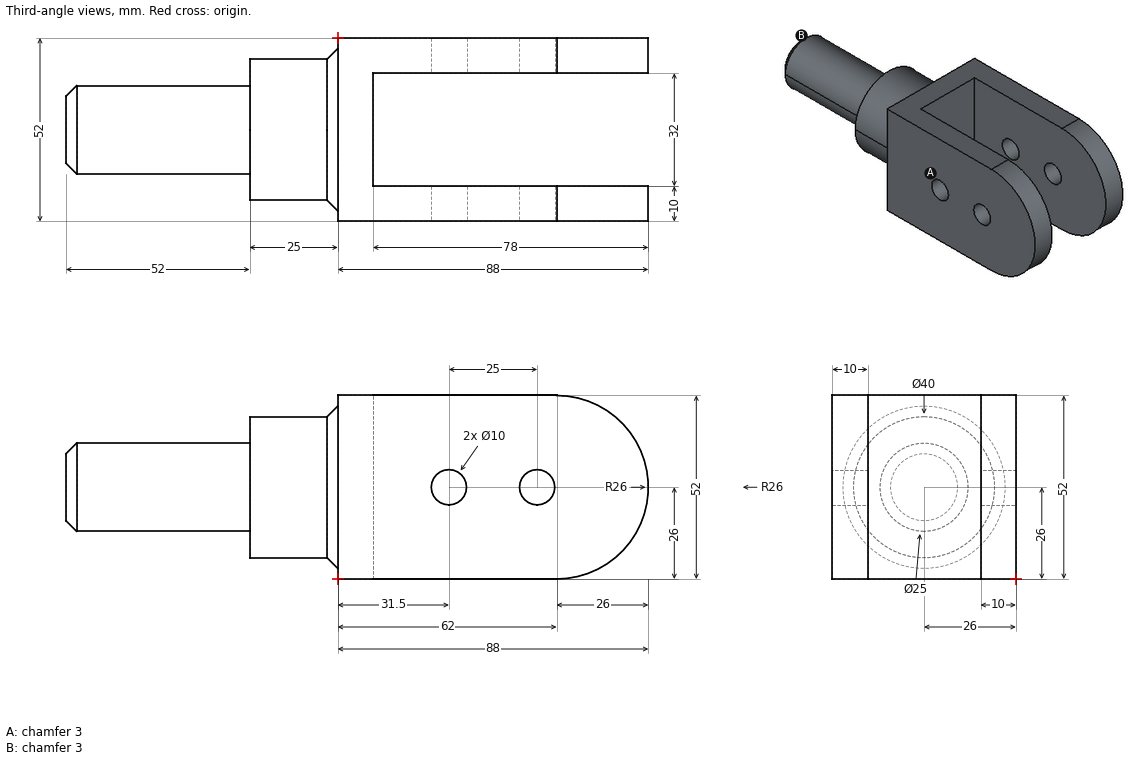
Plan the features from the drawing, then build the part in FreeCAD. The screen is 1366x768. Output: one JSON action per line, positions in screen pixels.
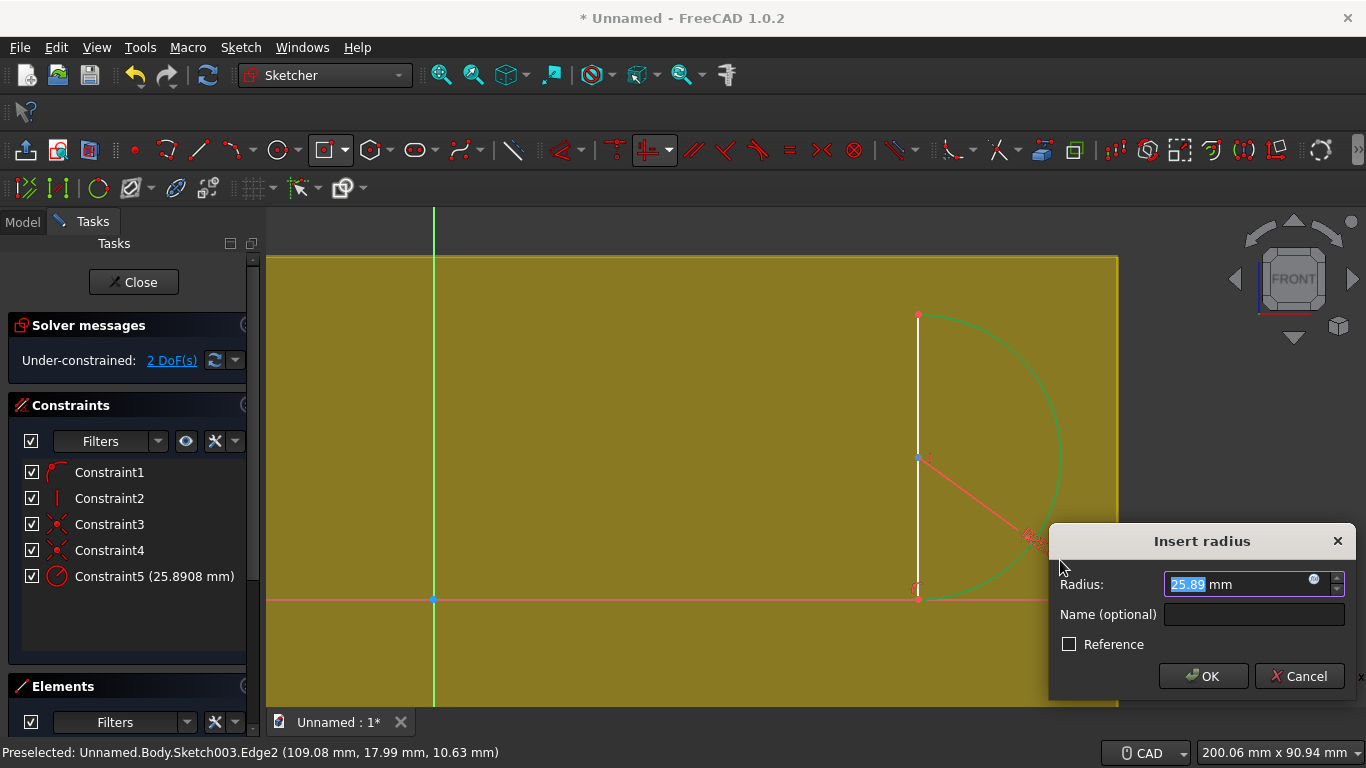
{"action": "type", "text": "26"}
{"action": "key", "text": "Return"}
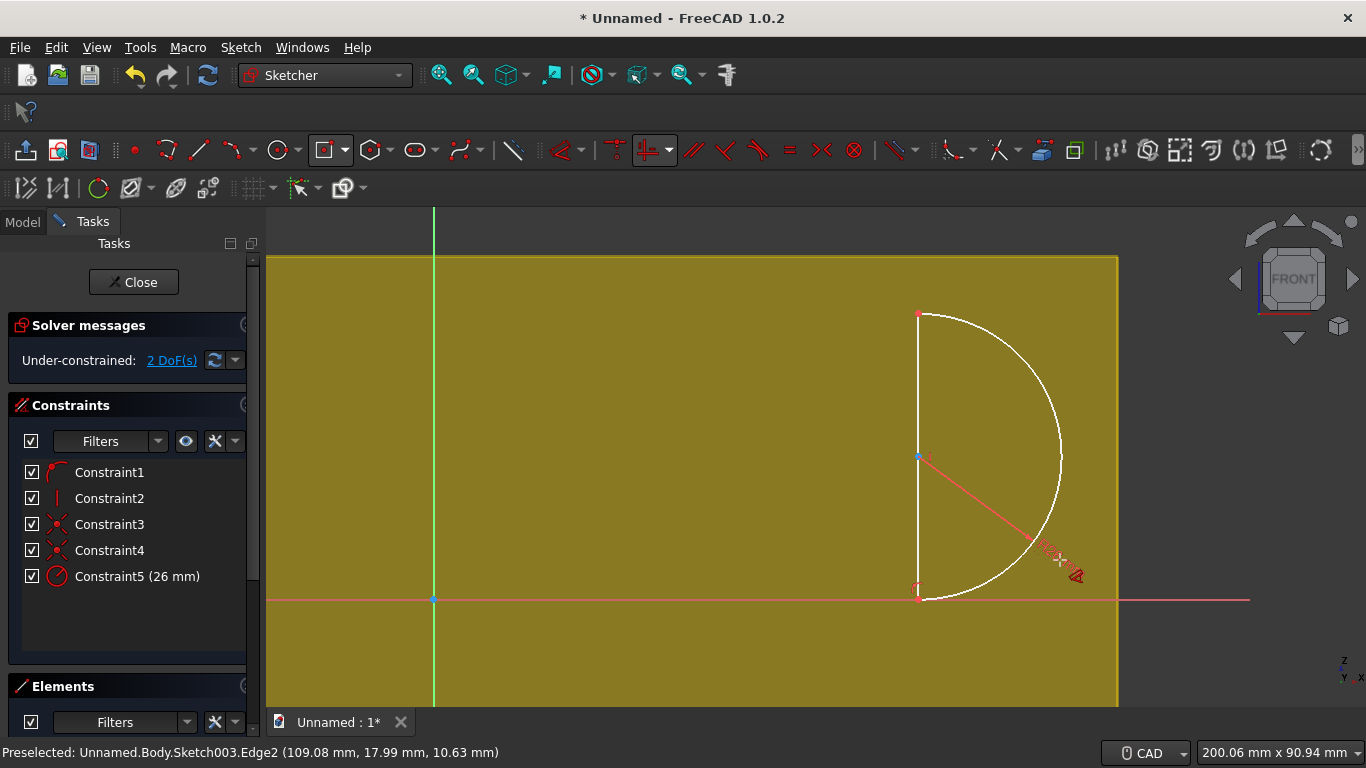
{"action": "left_click", "coordinate": [918, 314]}
{"action": "left_click", "coordinate": [676, 634]}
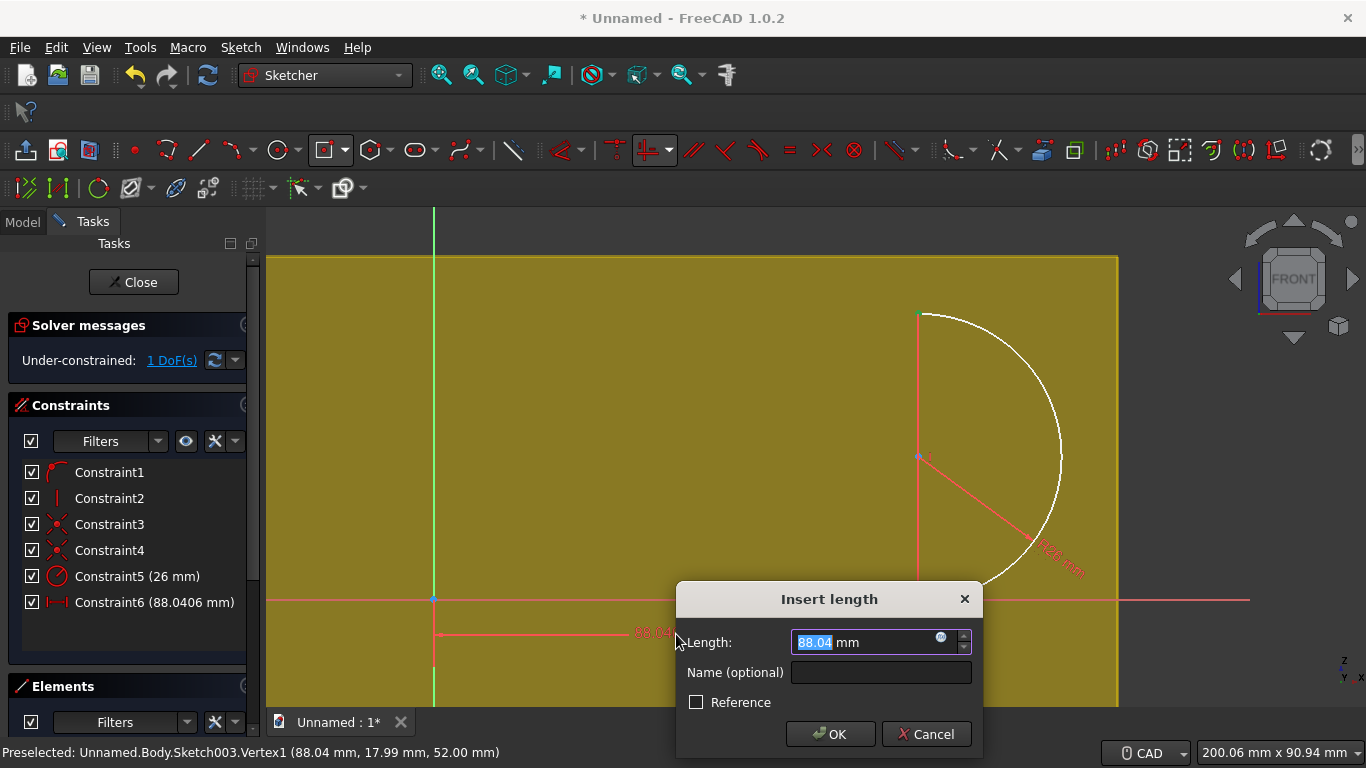
{"action": "type", "text": "88"}
{"action": "key", "text": "Return"}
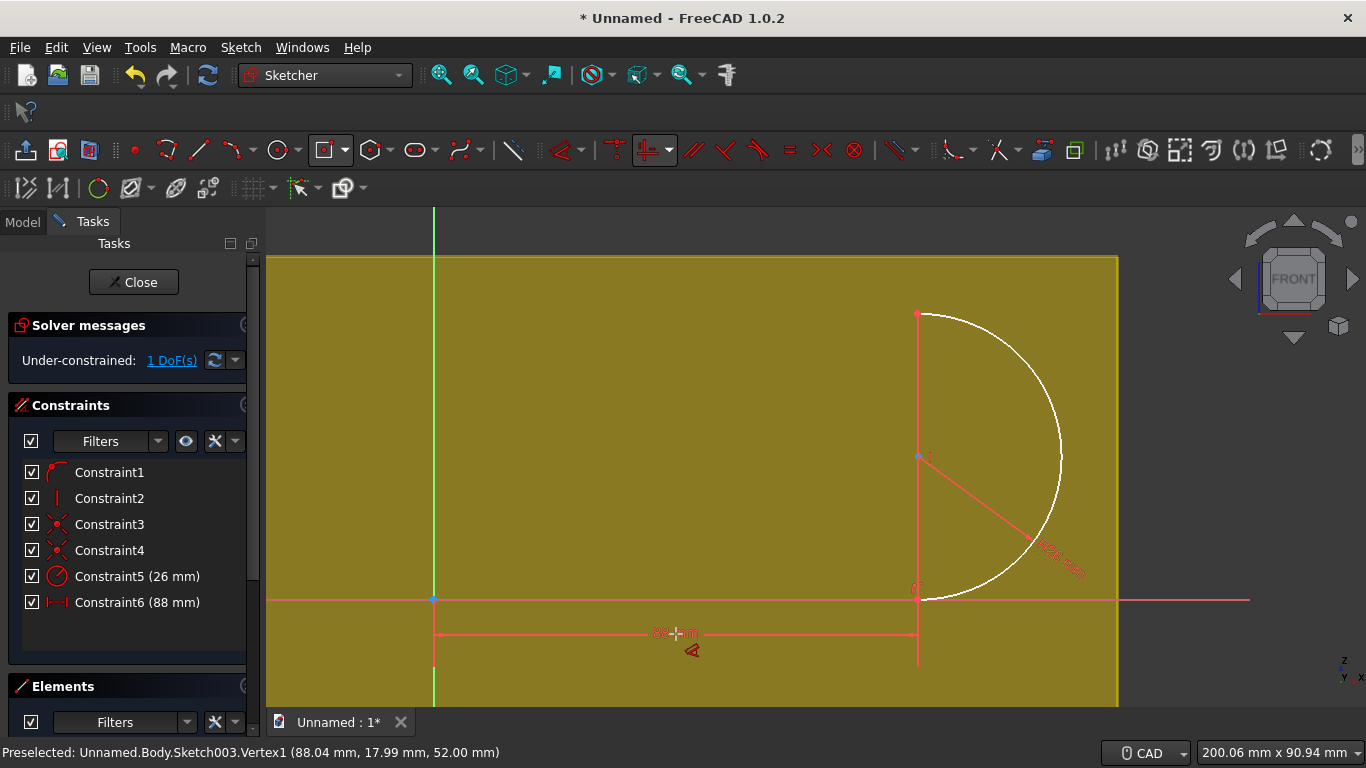
{"action": "left_click", "coordinate": [919, 457]}
{"action": "left_click", "coordinate": [565, 634]}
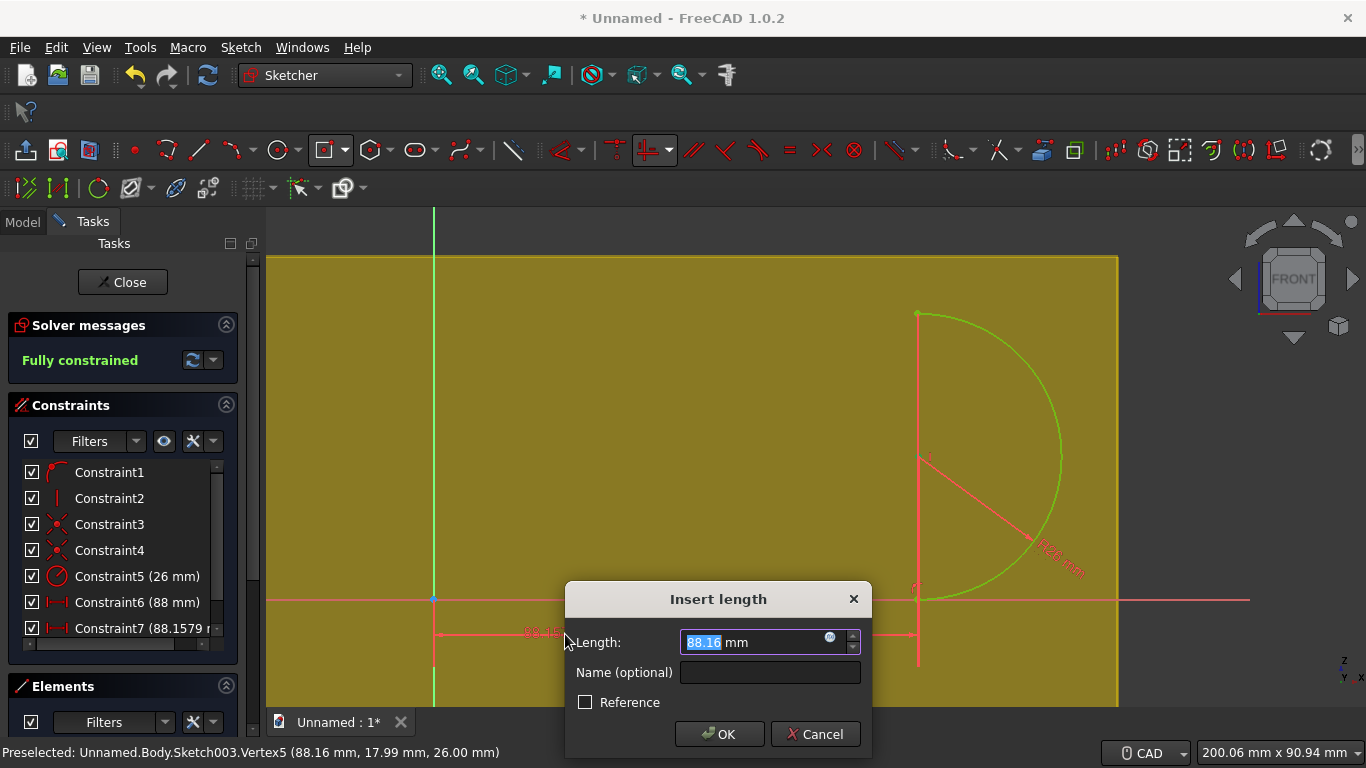
{"action": "type", "text": "88"}
{"action": "key", "text": "Return"}
{"action": "key", "text": "Escape"}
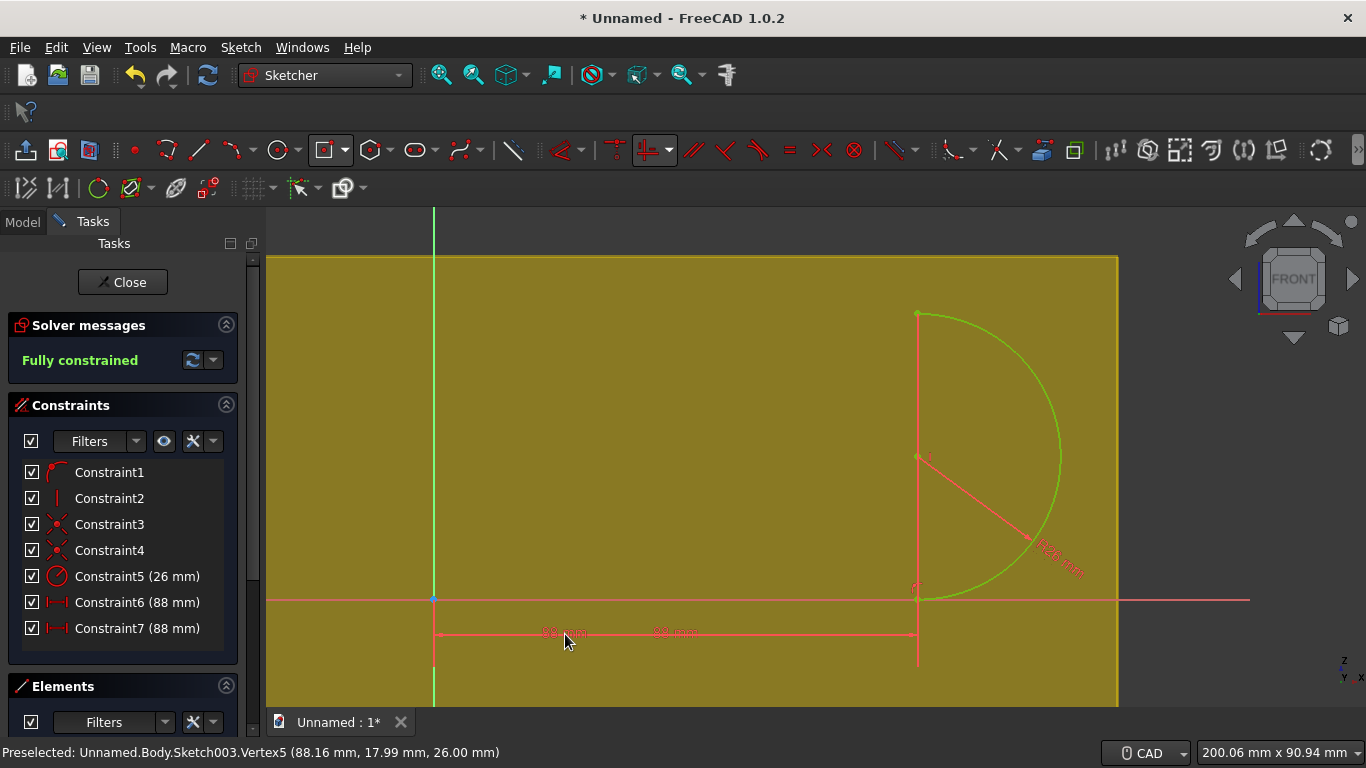
{"action": "left_click", "coordinate": [123, 282]}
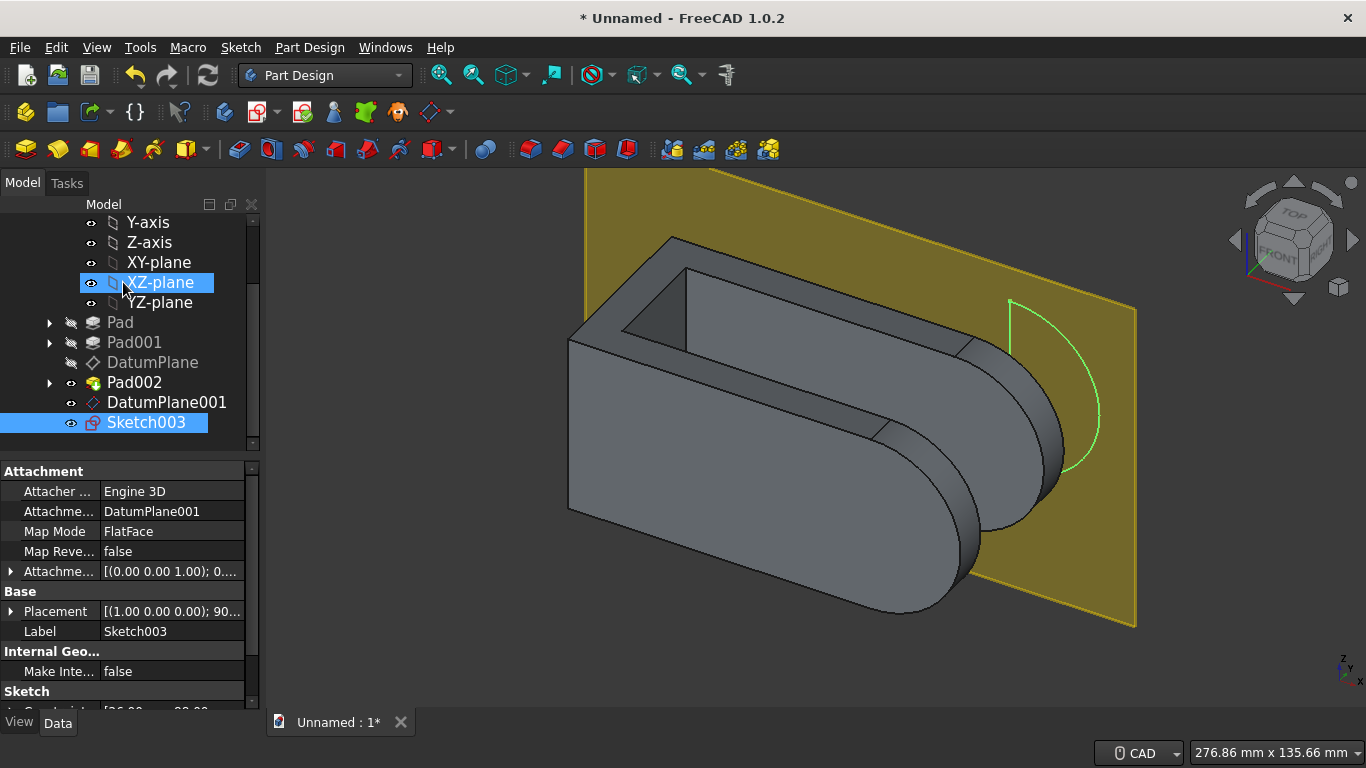
{"action": "left_click", "coordinate": [240, 150]}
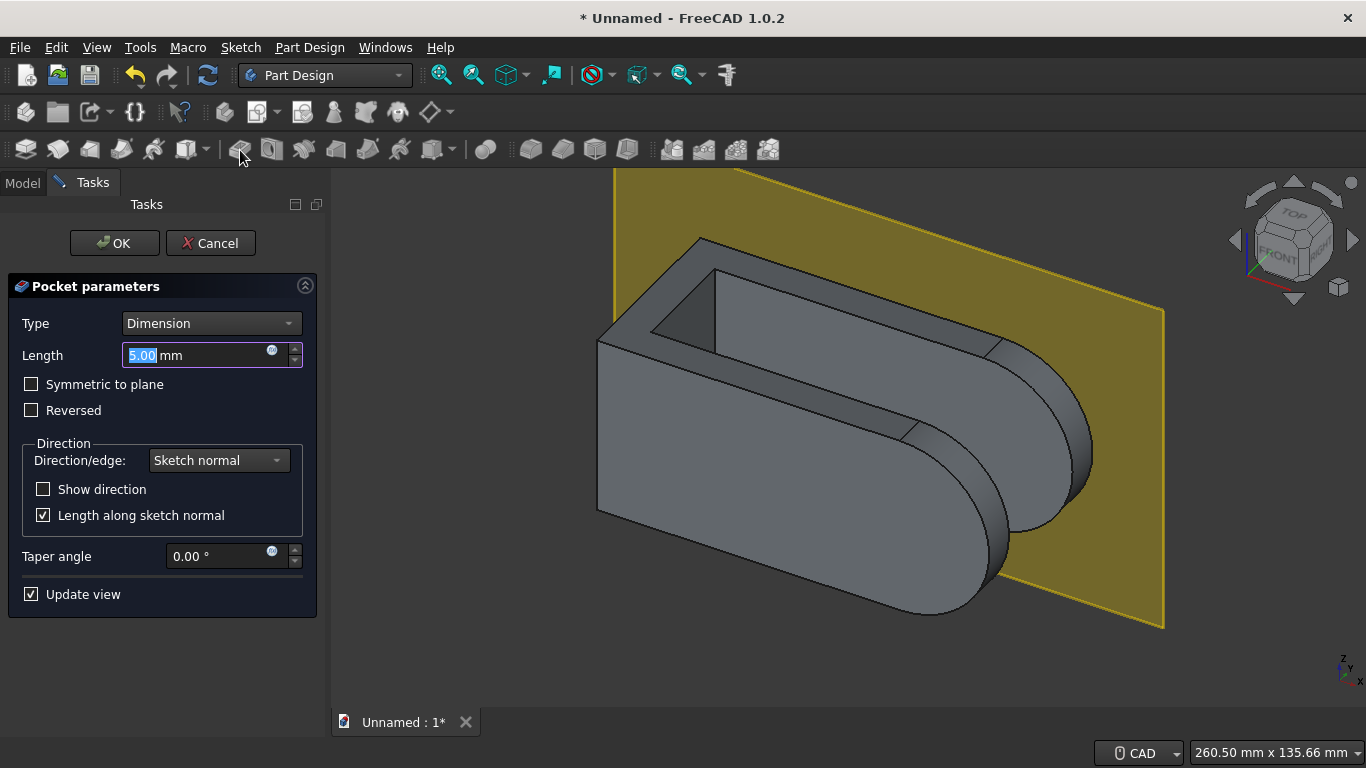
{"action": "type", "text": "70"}
{"action": "key", "text": "Tab"}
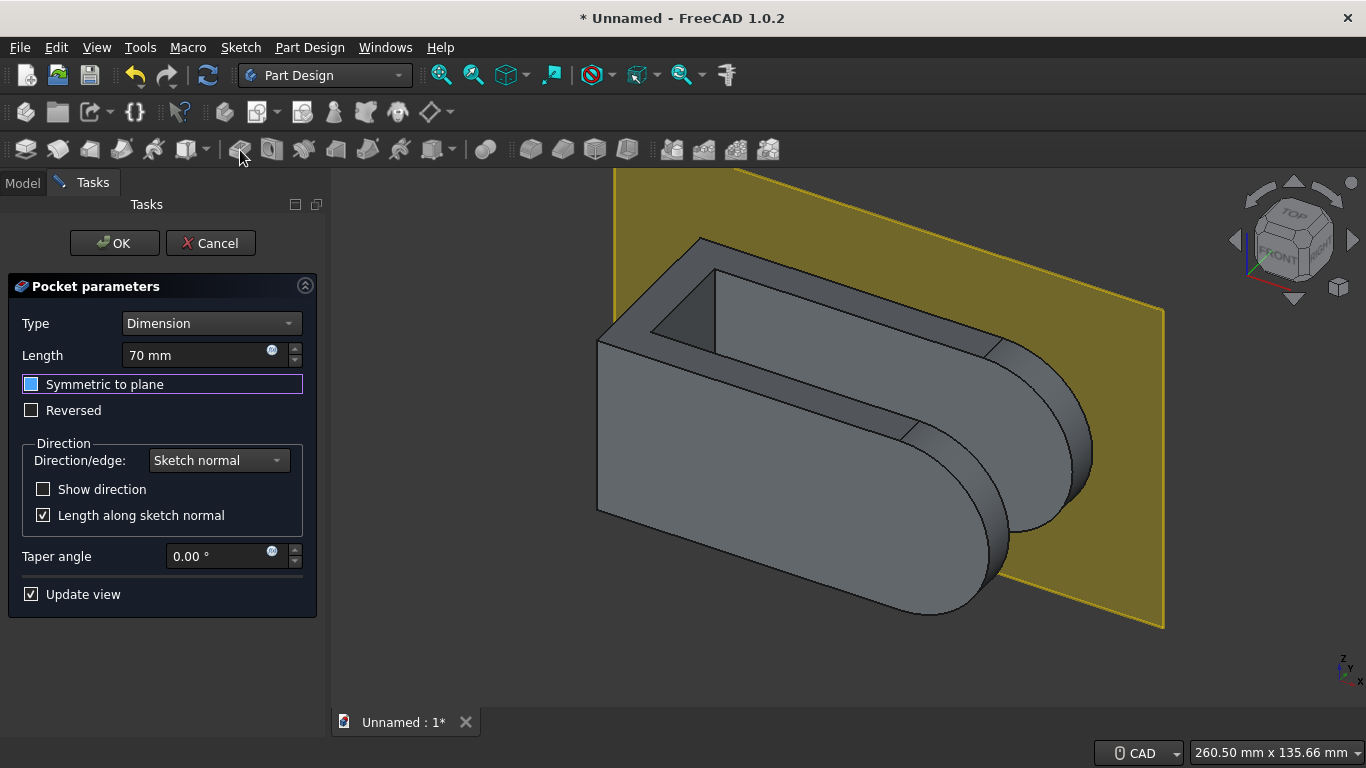
{"action": "left_click", "coordinate": [30, 410]}